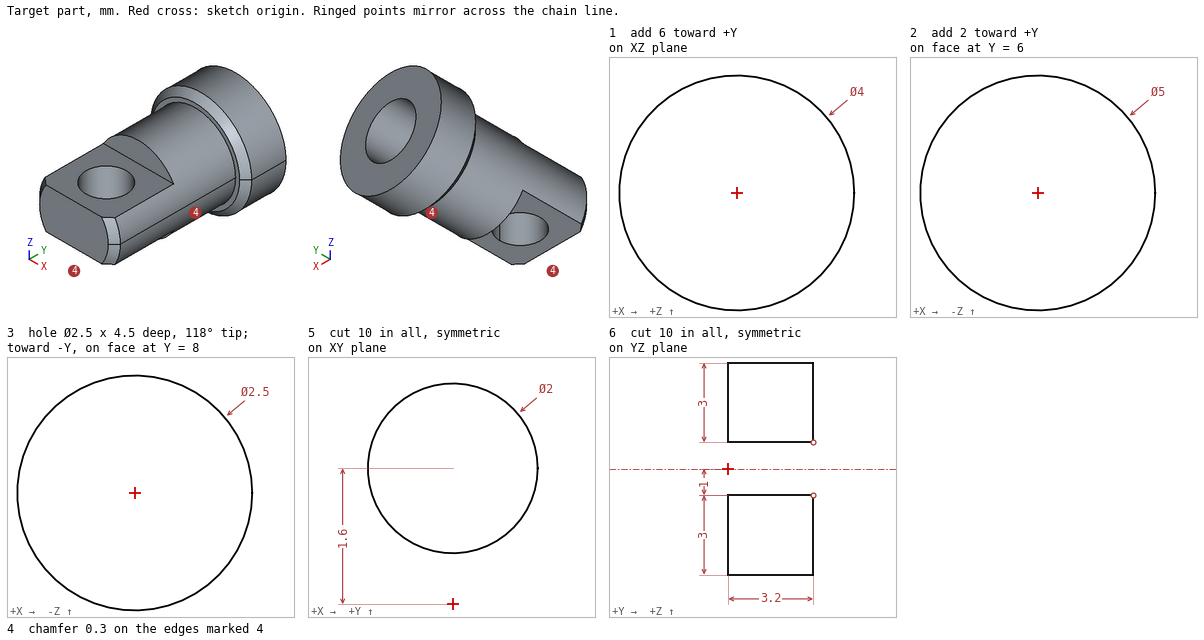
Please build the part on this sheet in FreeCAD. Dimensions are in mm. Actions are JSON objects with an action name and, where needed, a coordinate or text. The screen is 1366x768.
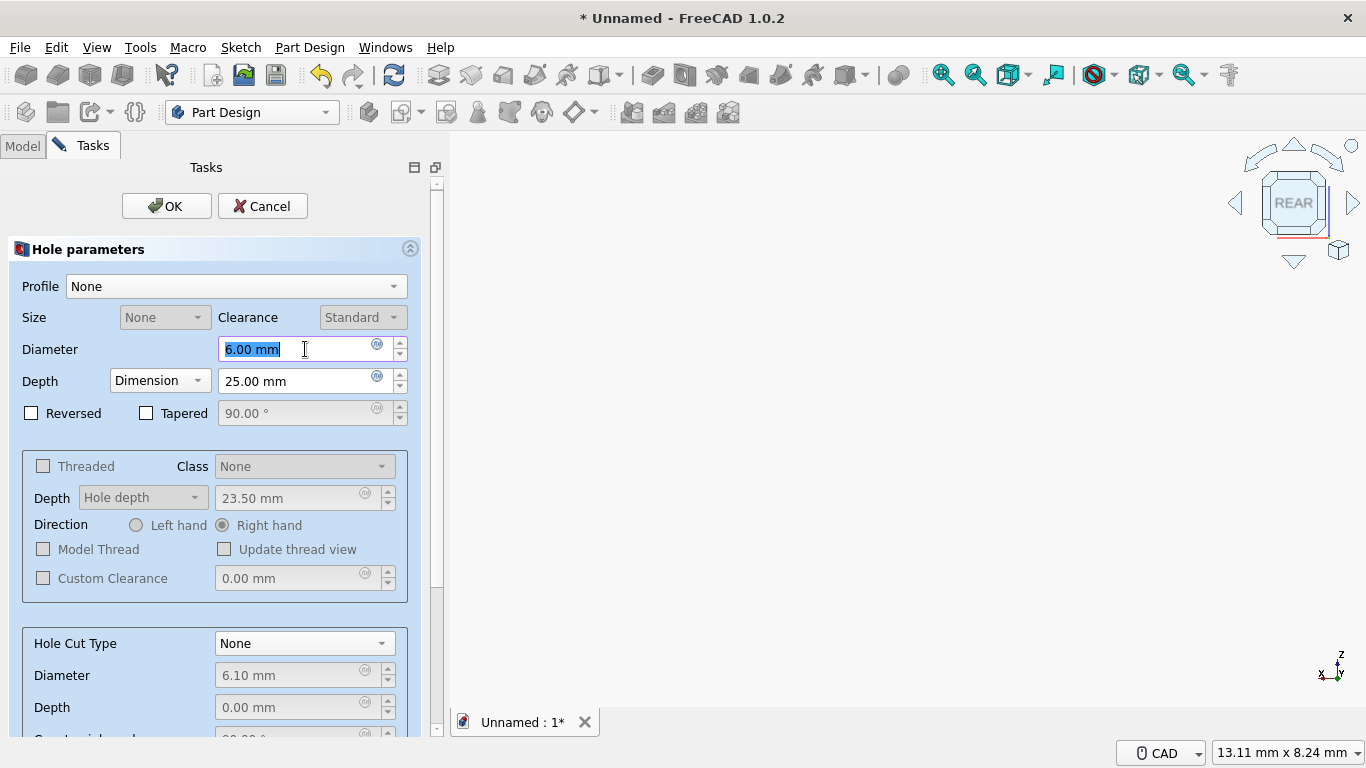
{"action": "type", "text": "2.5"}
{"action": "key", "text": "Tab"}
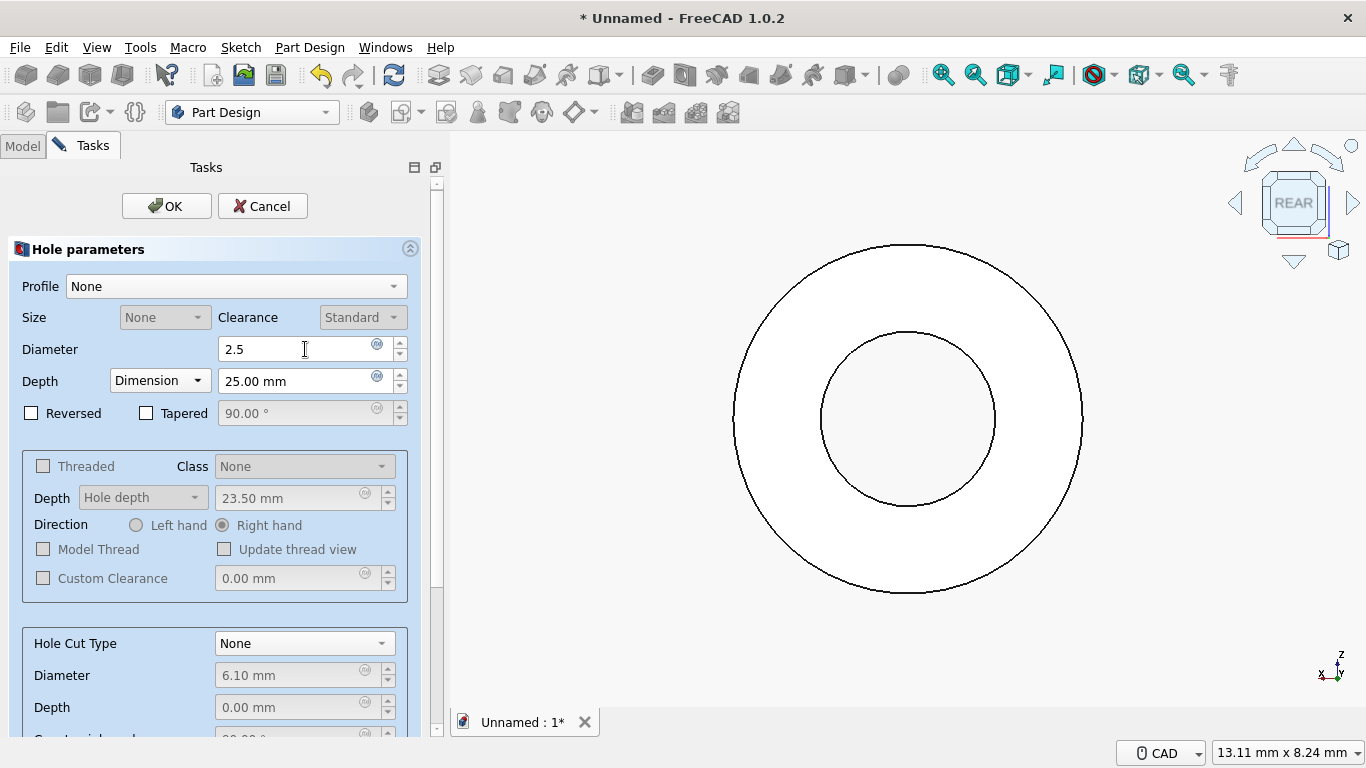
{"action": "triple_click", "coordinate": [305, 381]}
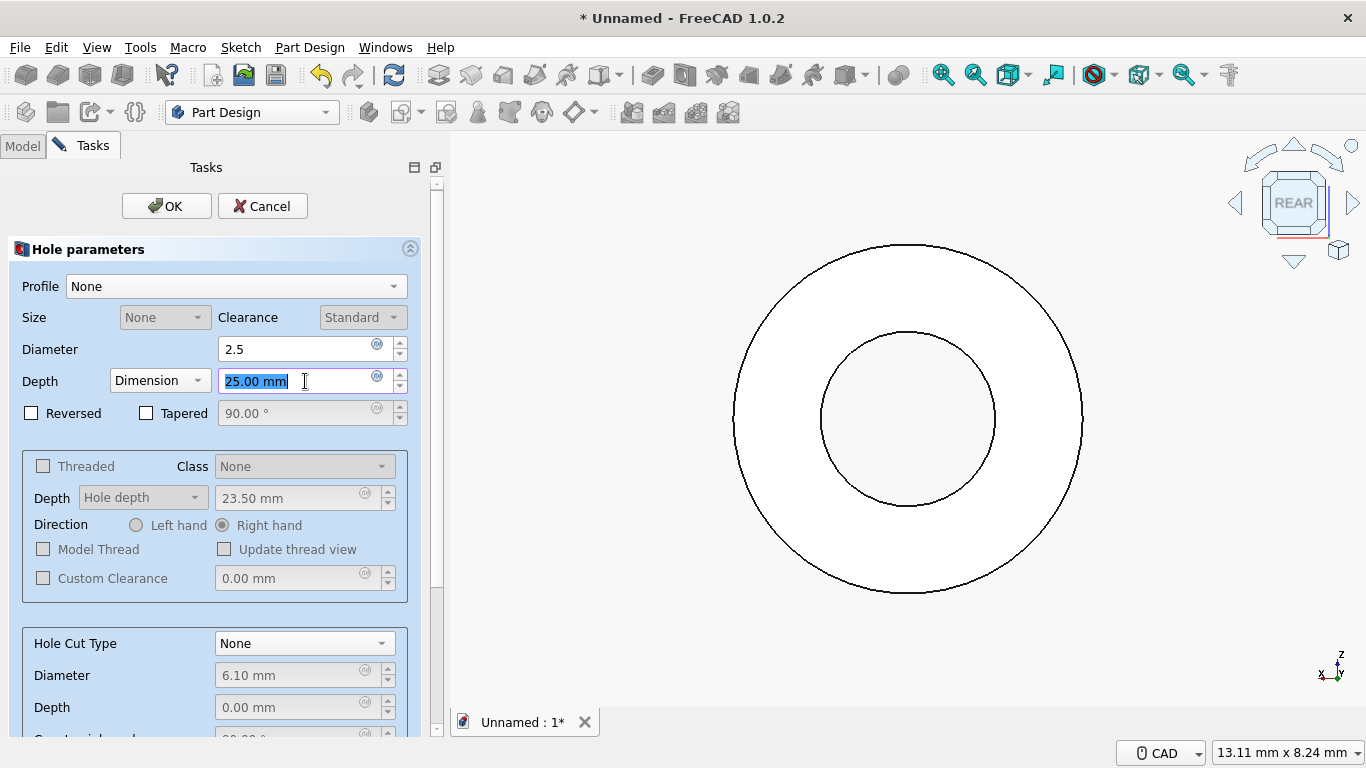
{"action": "type", "text": "4.5"}
{"action": "key", "text": "Tab"}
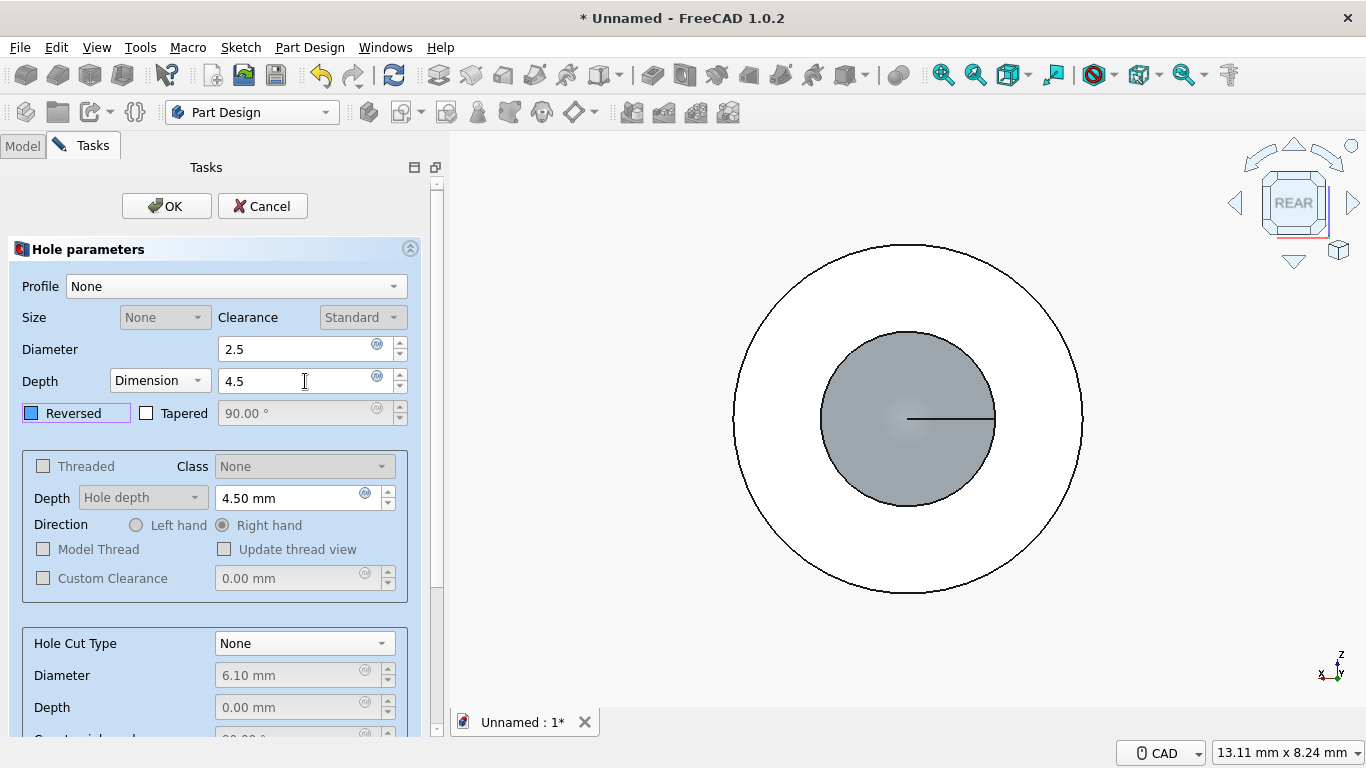
{"action": "left_click", "coordinate": [167, 206]}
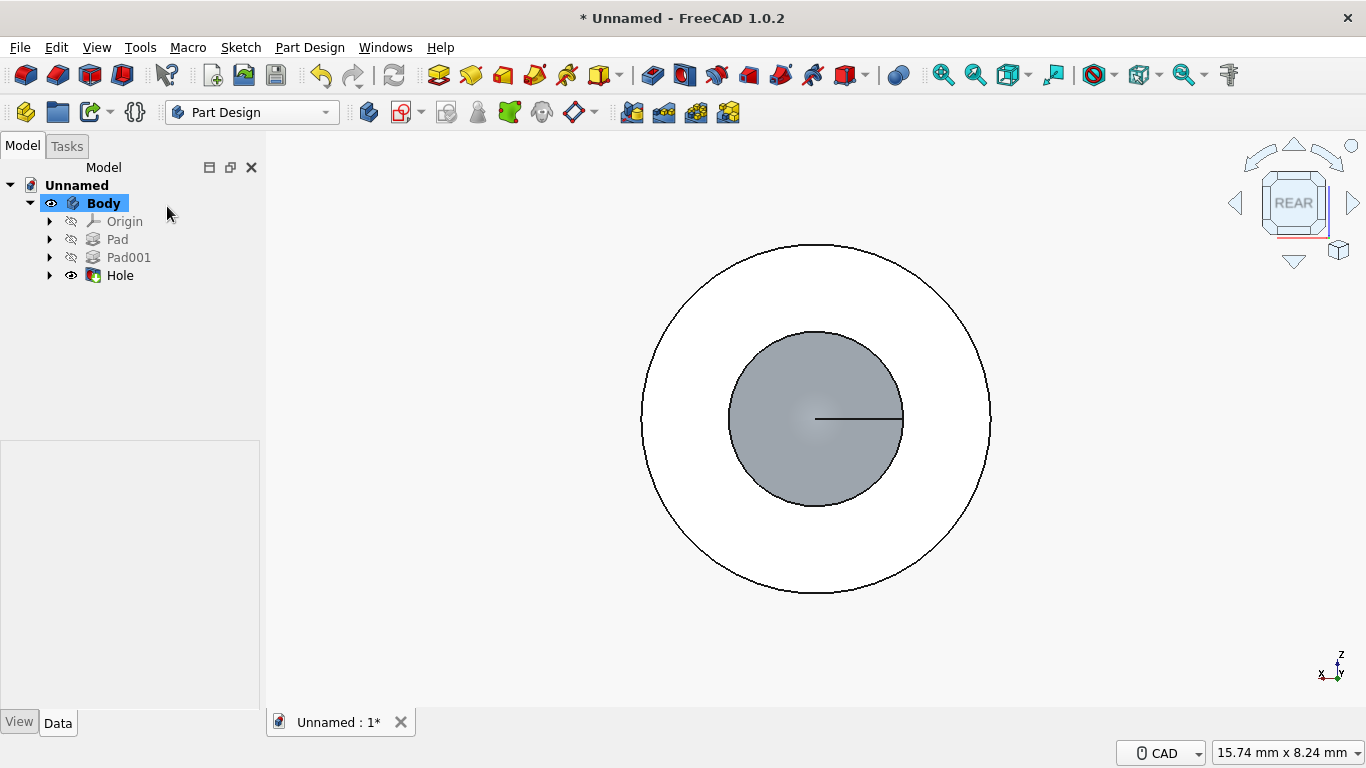
{"action": "key", "text": "0"}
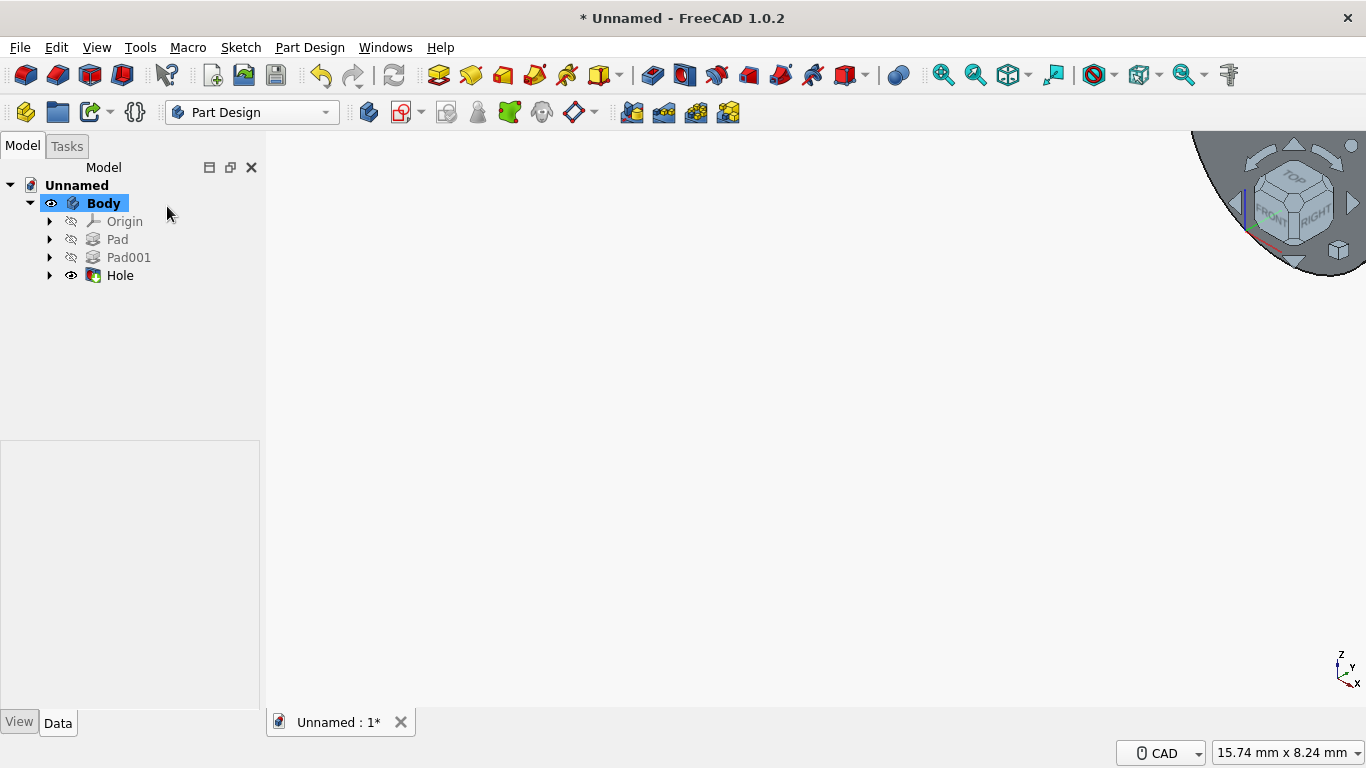
{"action": "left_click", "coordinate": [944, 76]}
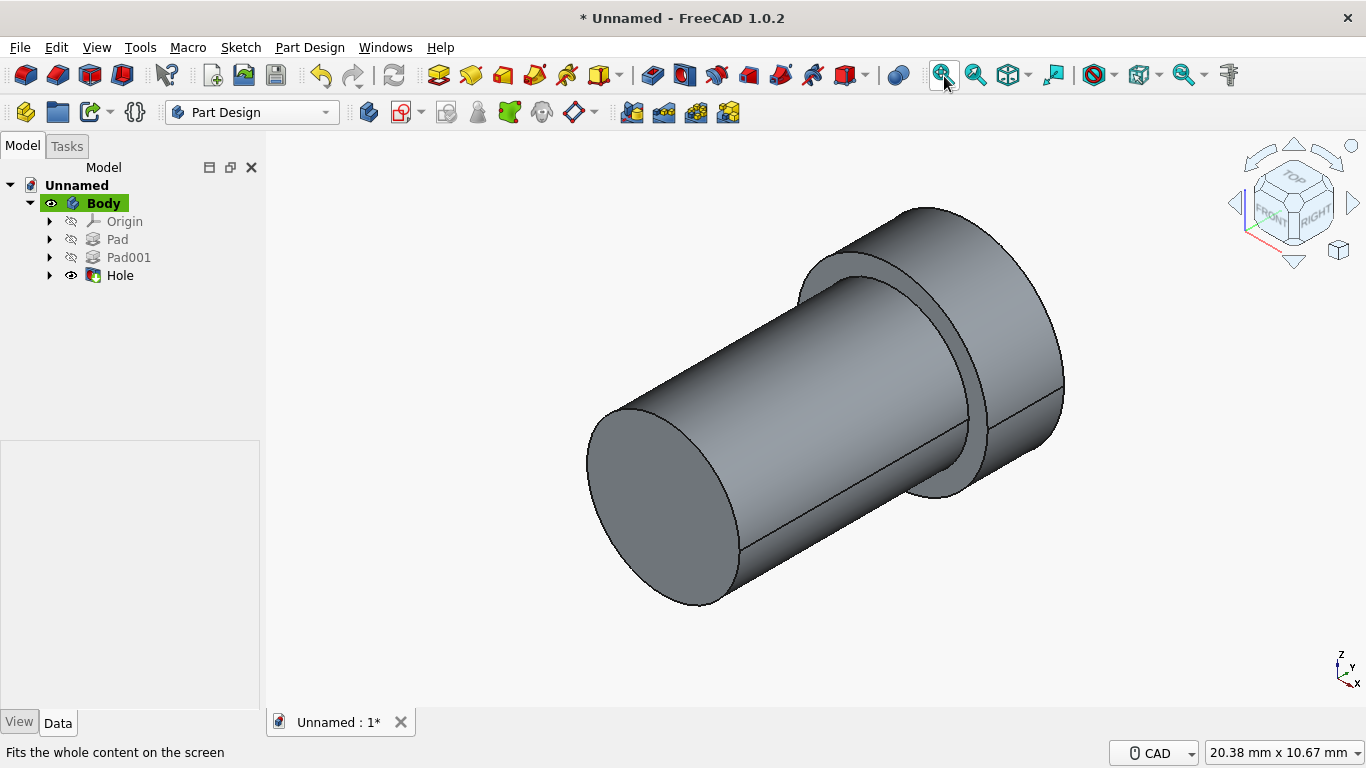
{"action": "left_click", "coordinate": [640, 409]}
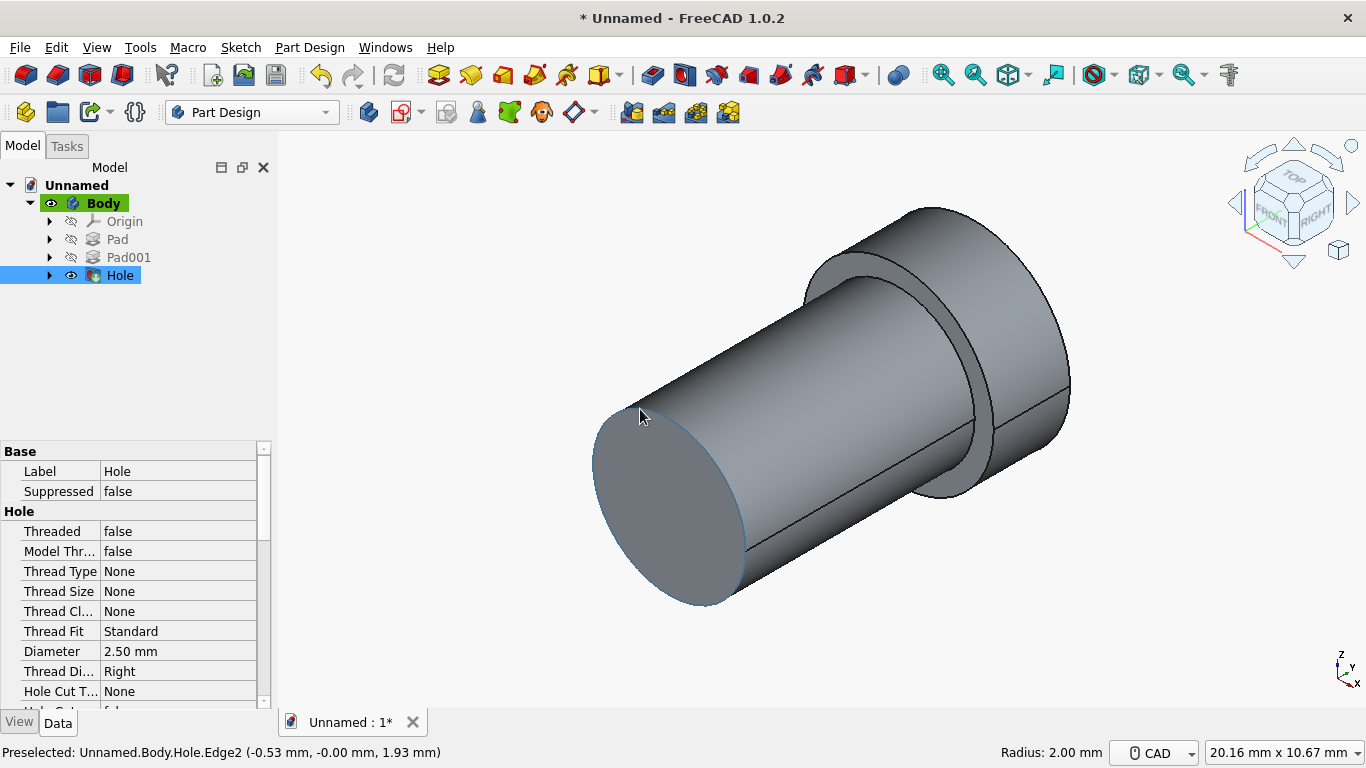
{"action": "left_click", "coordinate": [869, 252], "text": "ctrl"}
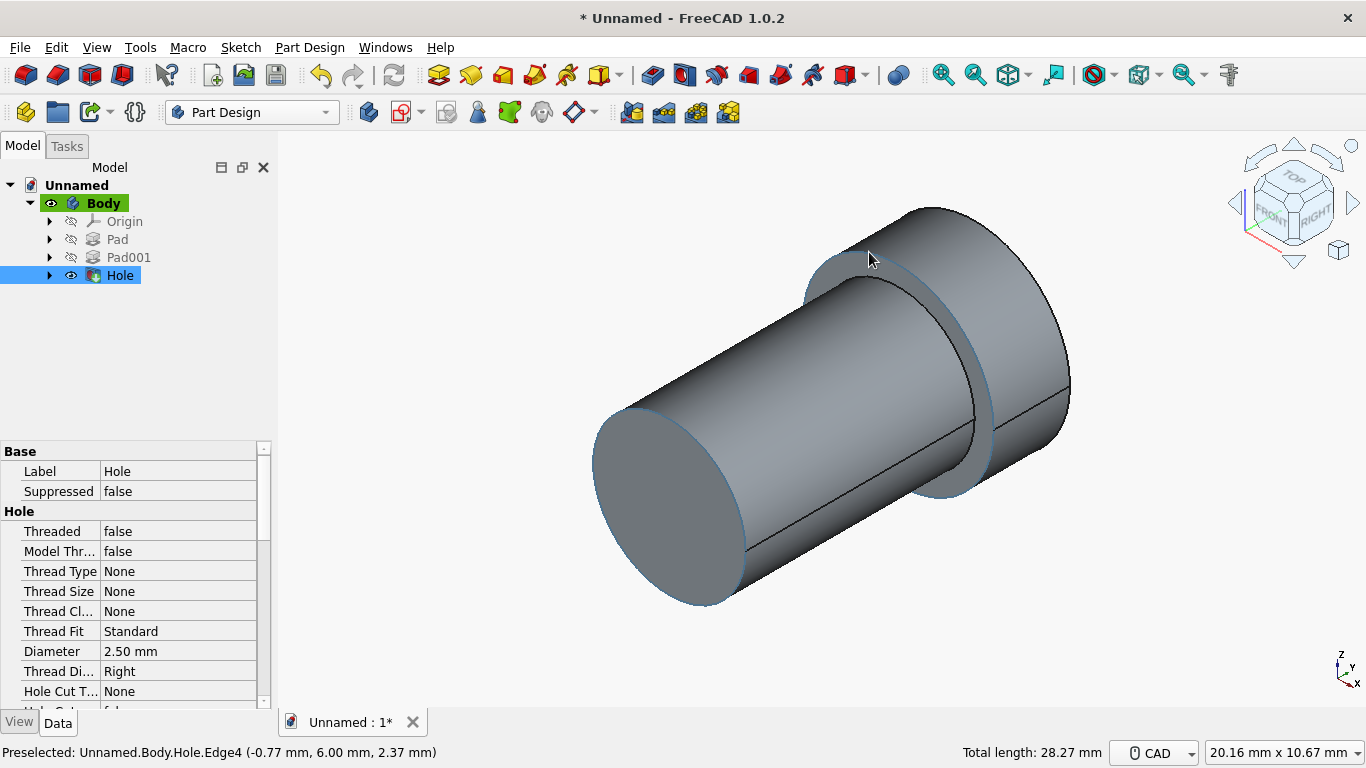
{"action": "left_click", "coordinate": [58, 76]}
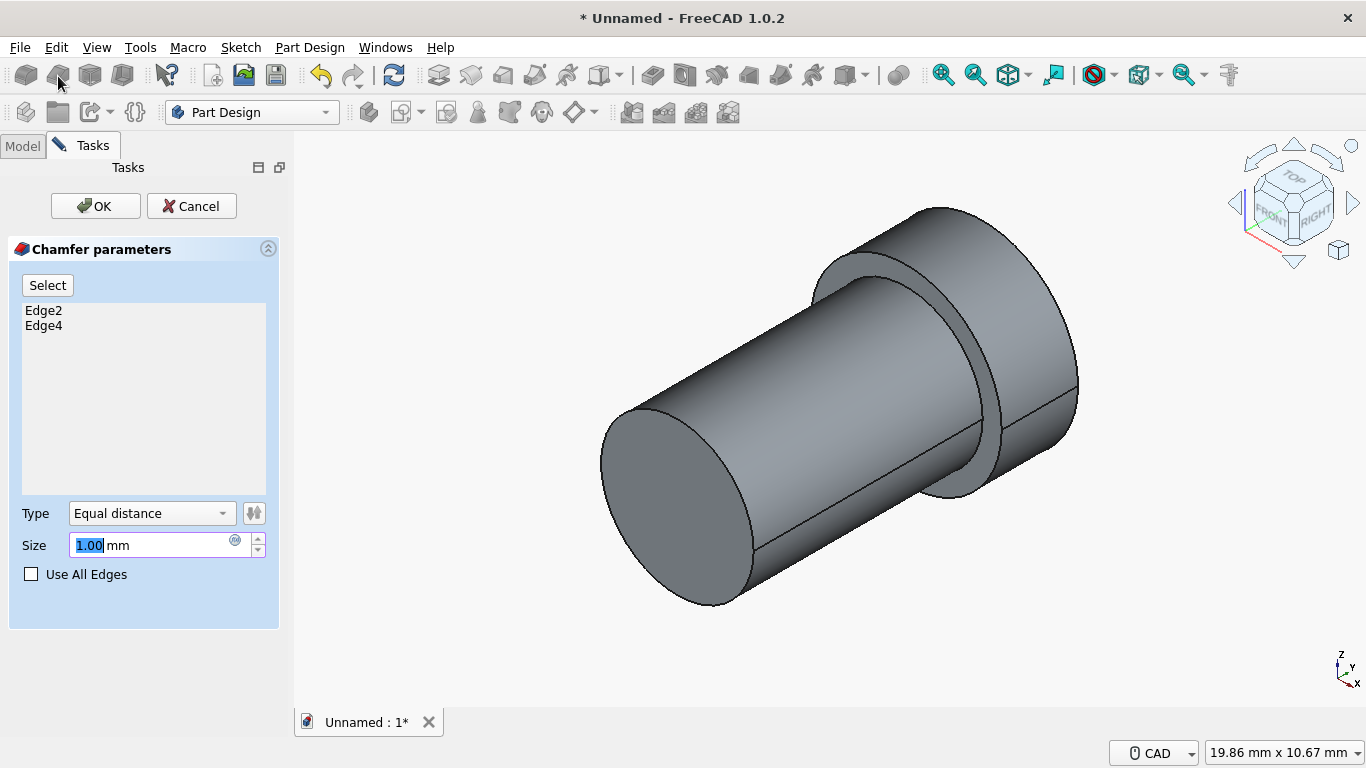
{"action": "type", "text": "0.3"}
{"action": "key", "text": "Tab"}